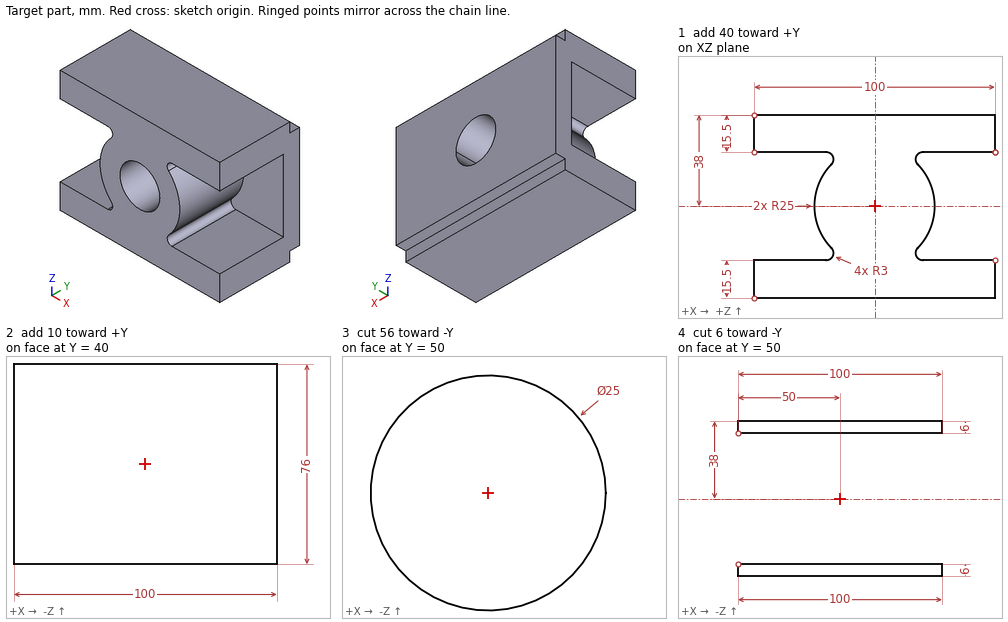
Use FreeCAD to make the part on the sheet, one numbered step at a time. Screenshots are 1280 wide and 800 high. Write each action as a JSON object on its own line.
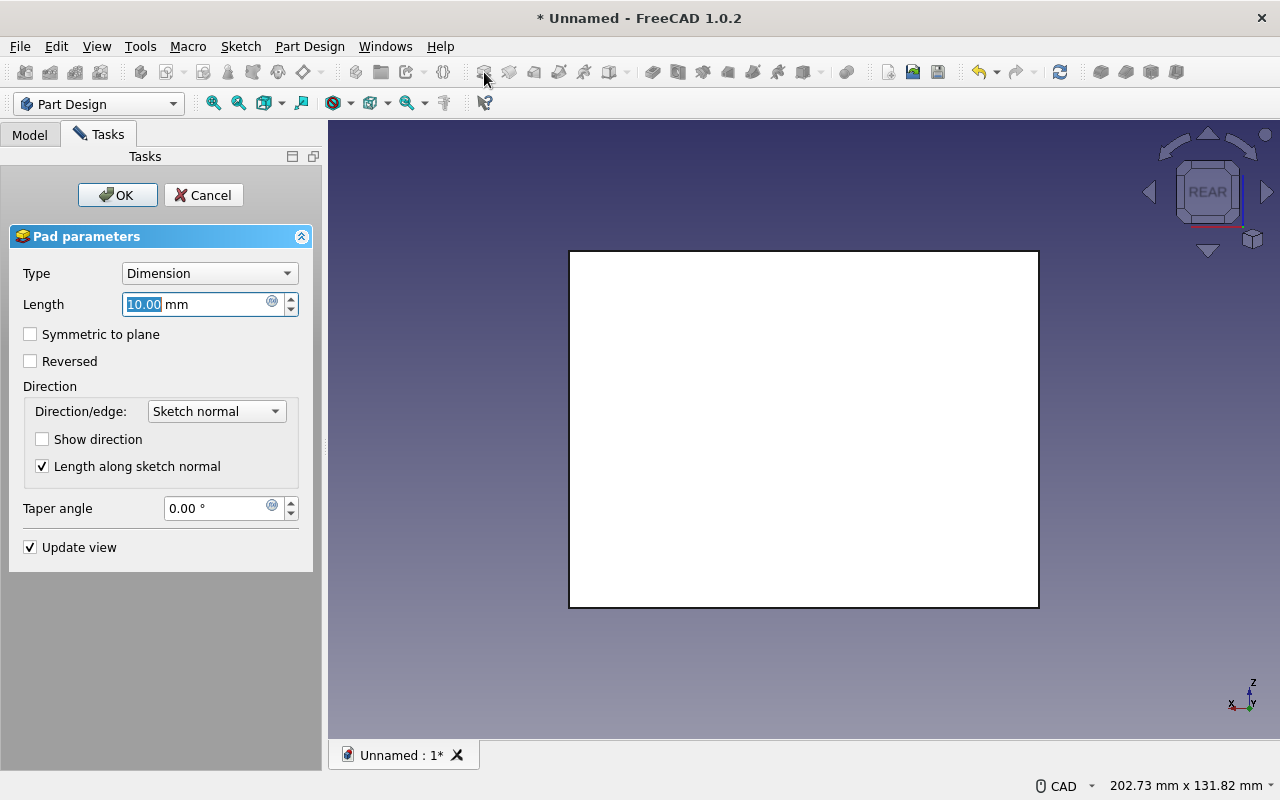
{"action": "type", "text": "10"}
{"action": "key", "text": "Tab"}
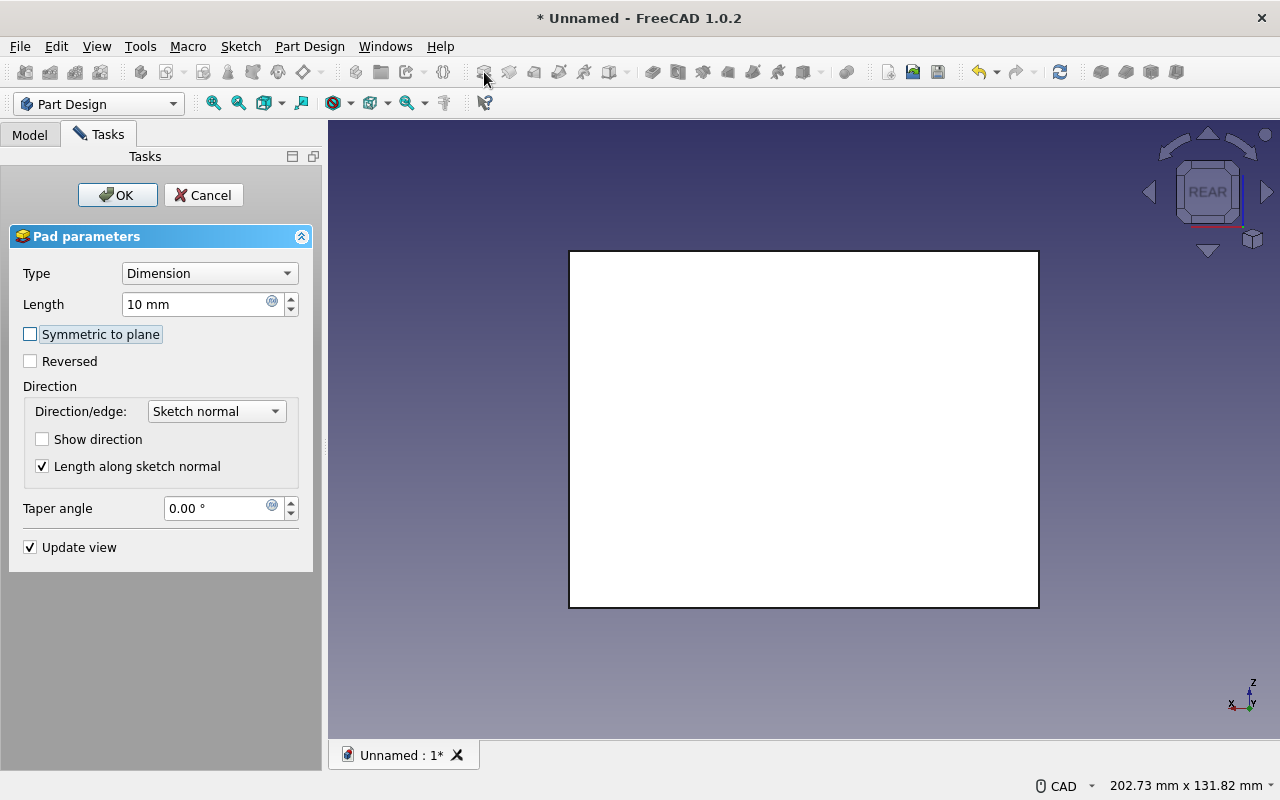
{"action": "left_click", "coordinate": [118, 195]}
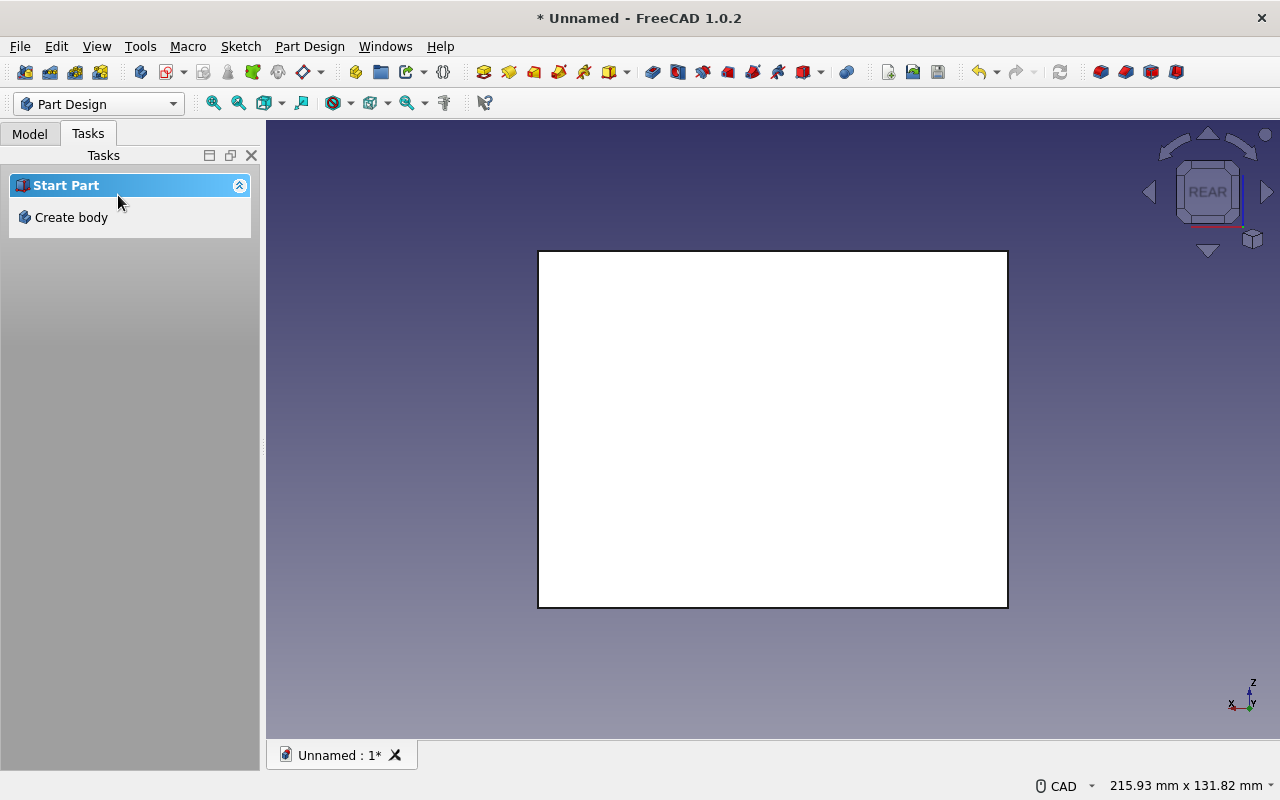
{"action": "left_click", "coordinate": [773, 428]}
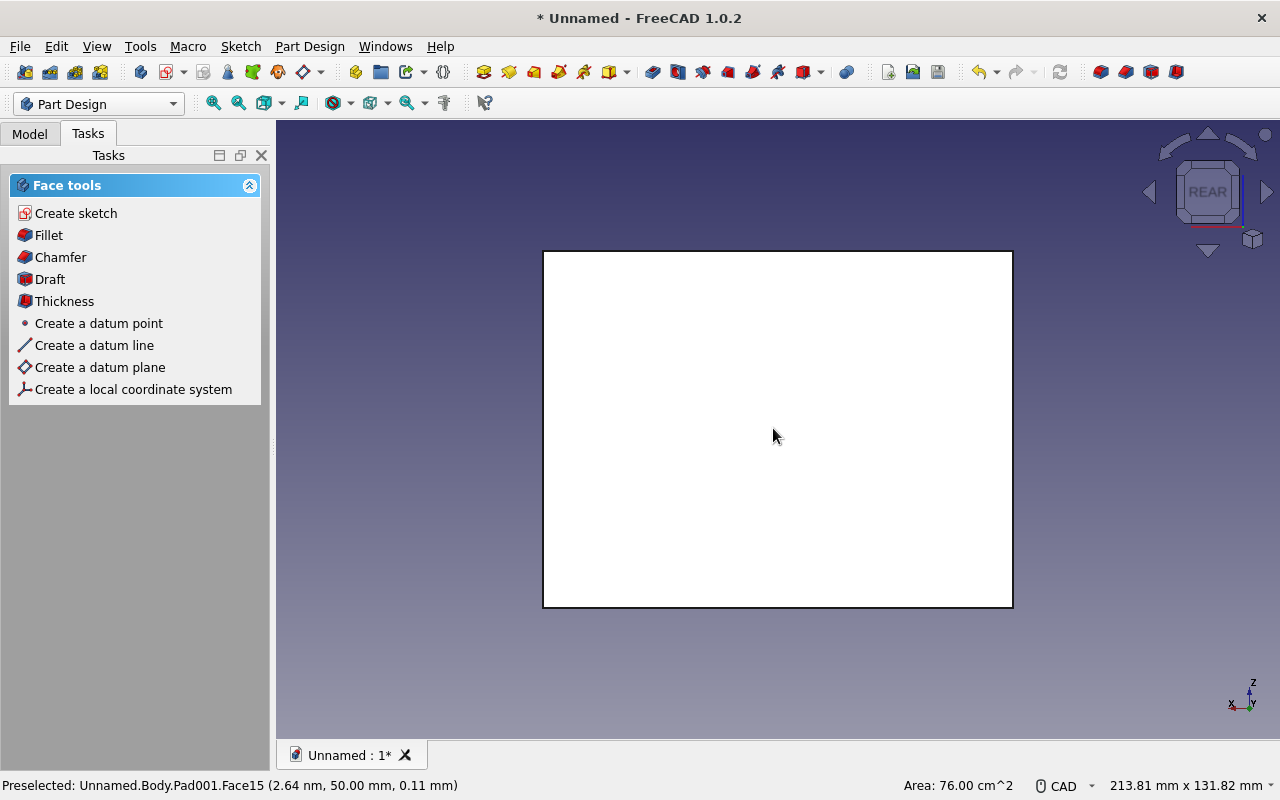
{"action": "left_click", "coordinate": [166, 72]}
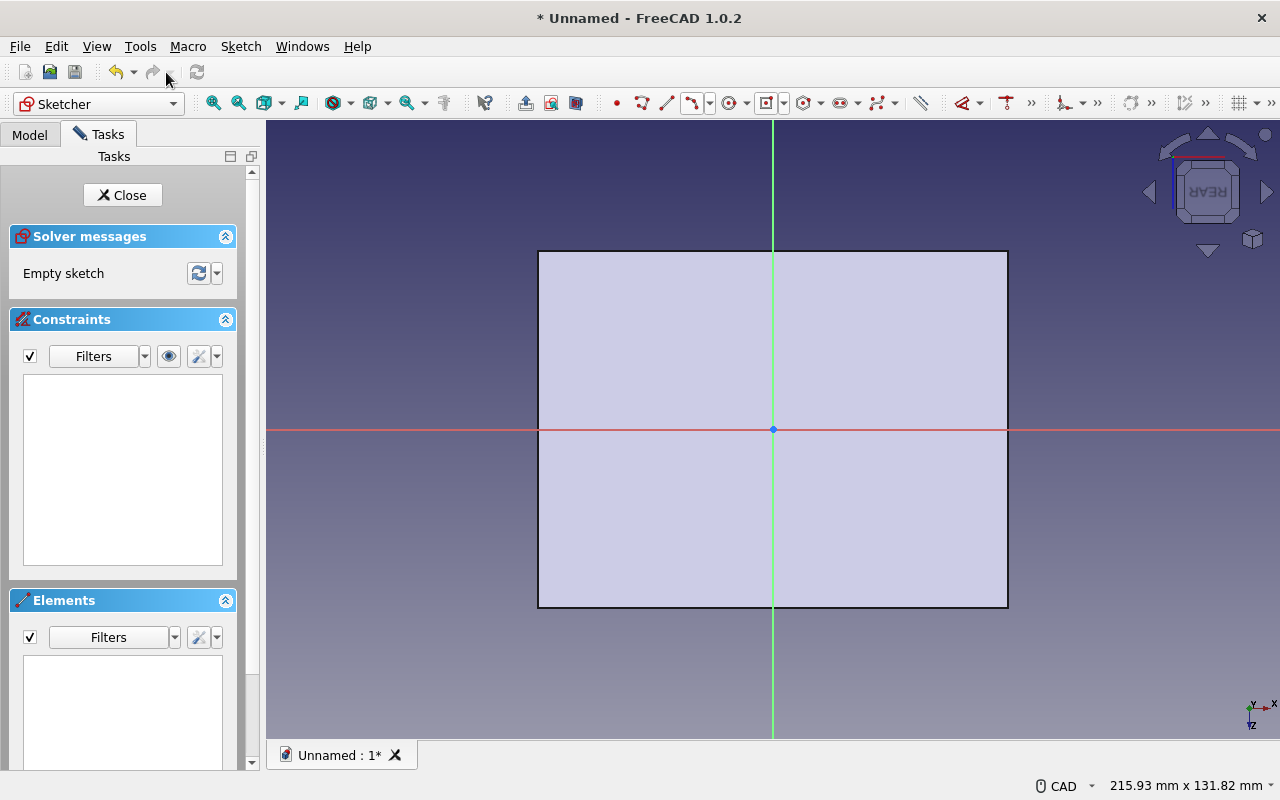
{"action": "scroll", "coordinate": [803, 429], "scroll_direction": "up", "scroll_amount": 6}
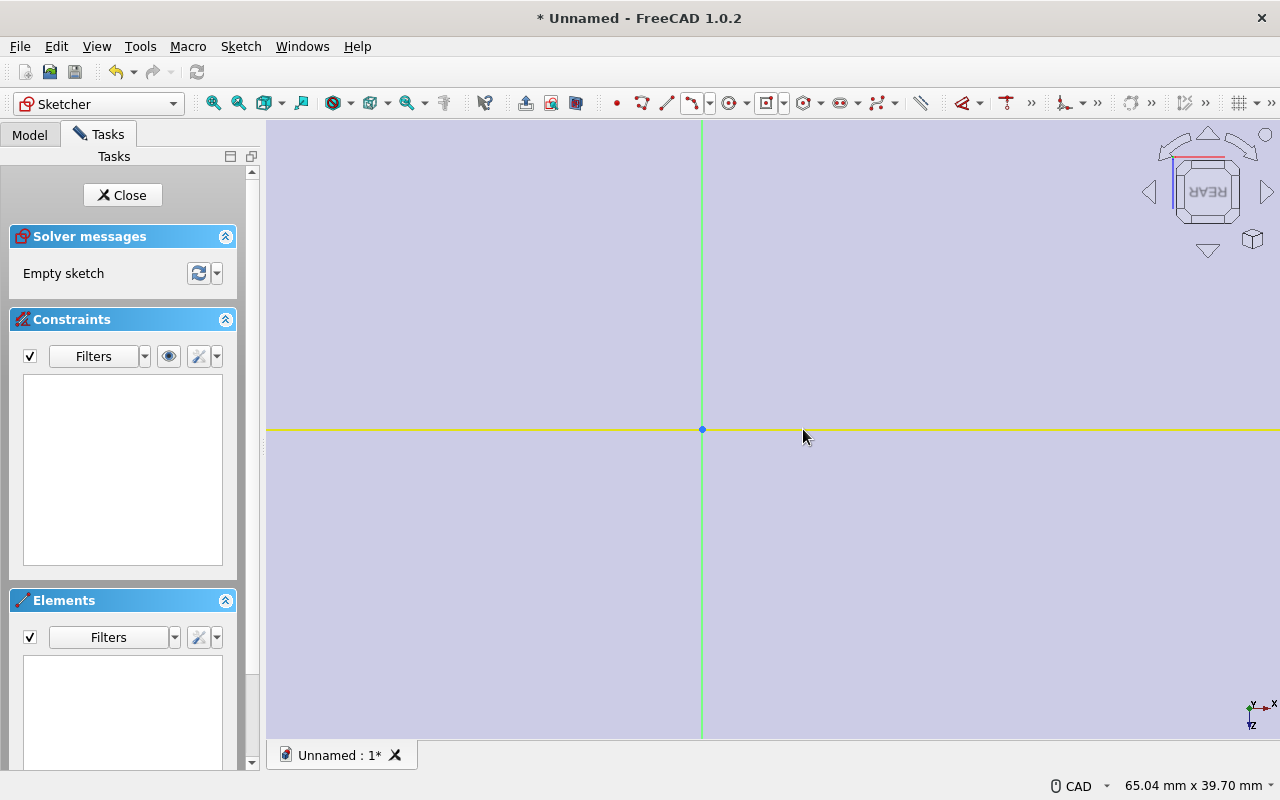
{"action": "left_click", "coordinate": [728, 104]}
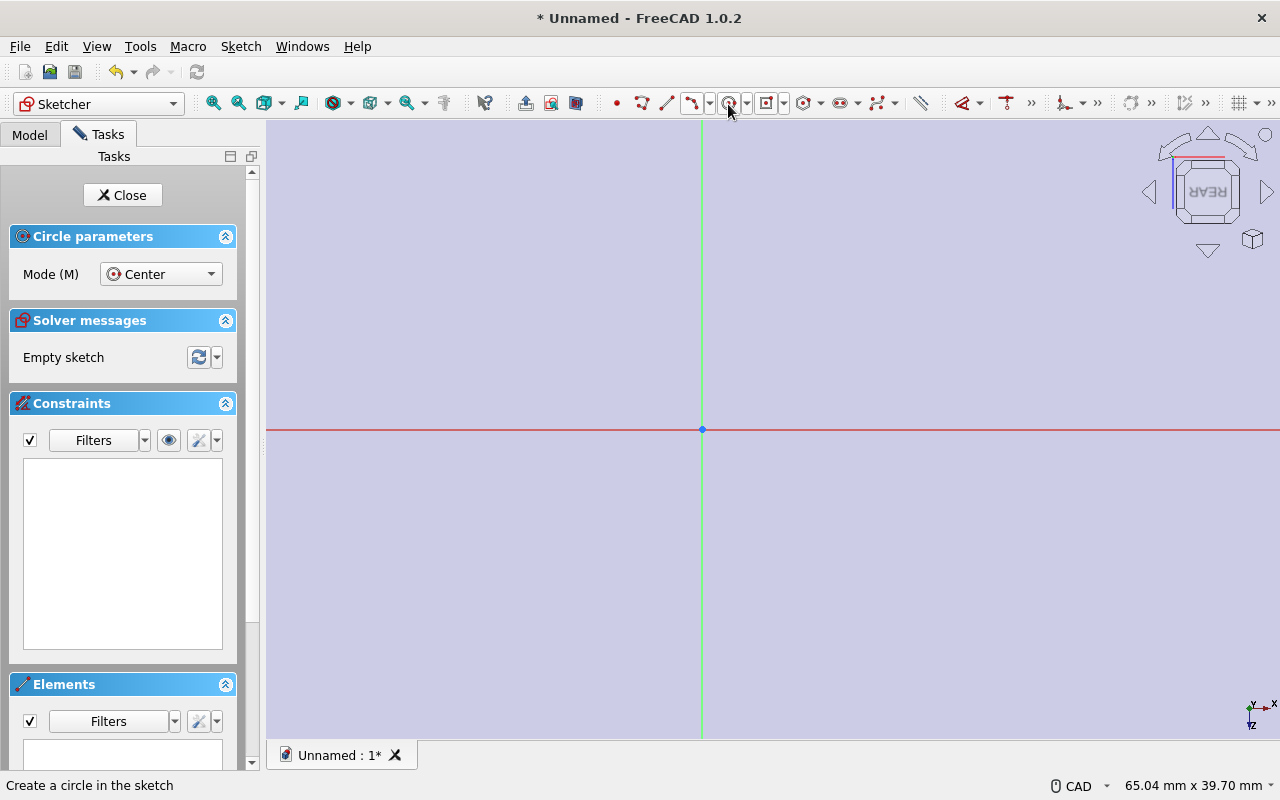
{"action": "left_click", "coordinate": [702, 429]}
{"action": "mouse_move", "coordinate": [840, 292]}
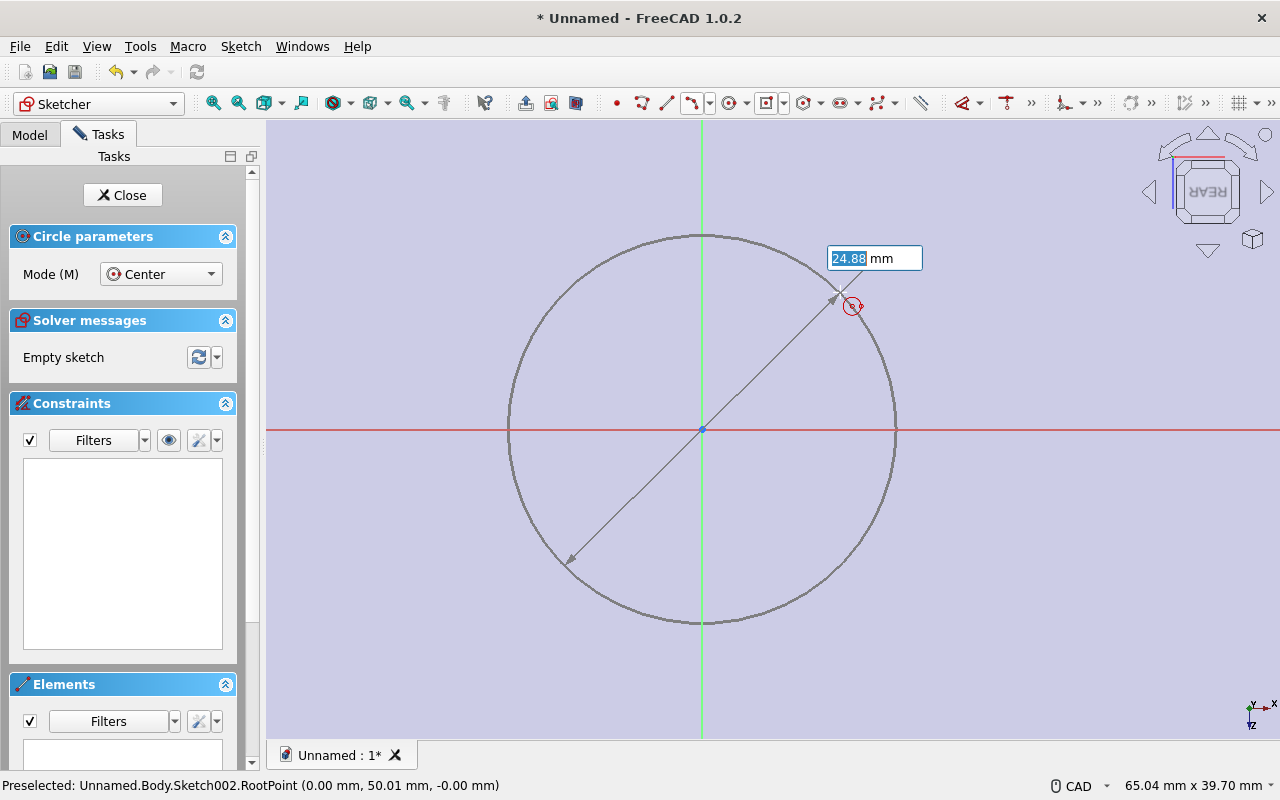
{"action": "type", "text": "25"}
{"action": "key", "text": "Return"}
{"action": "key", "text": "Escape"}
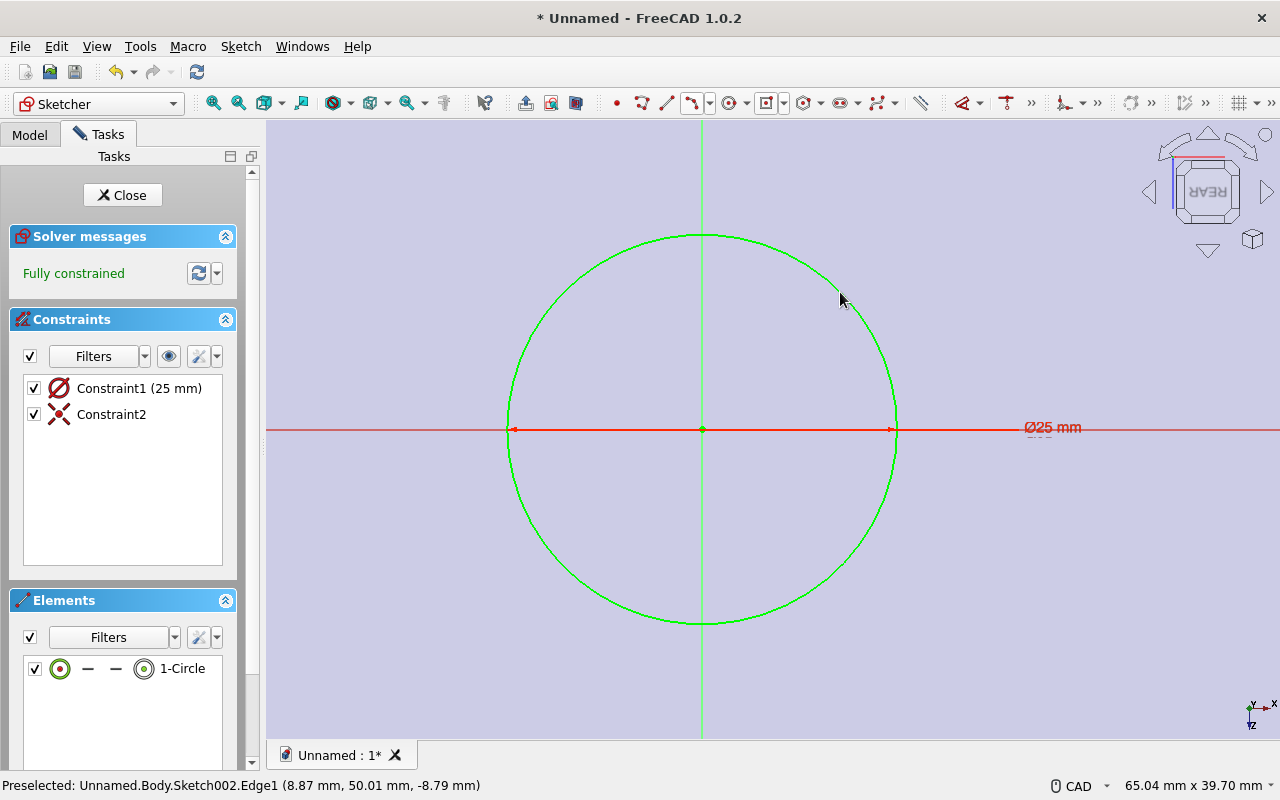
{"action": "left_click", "coordinate": [123, 195]}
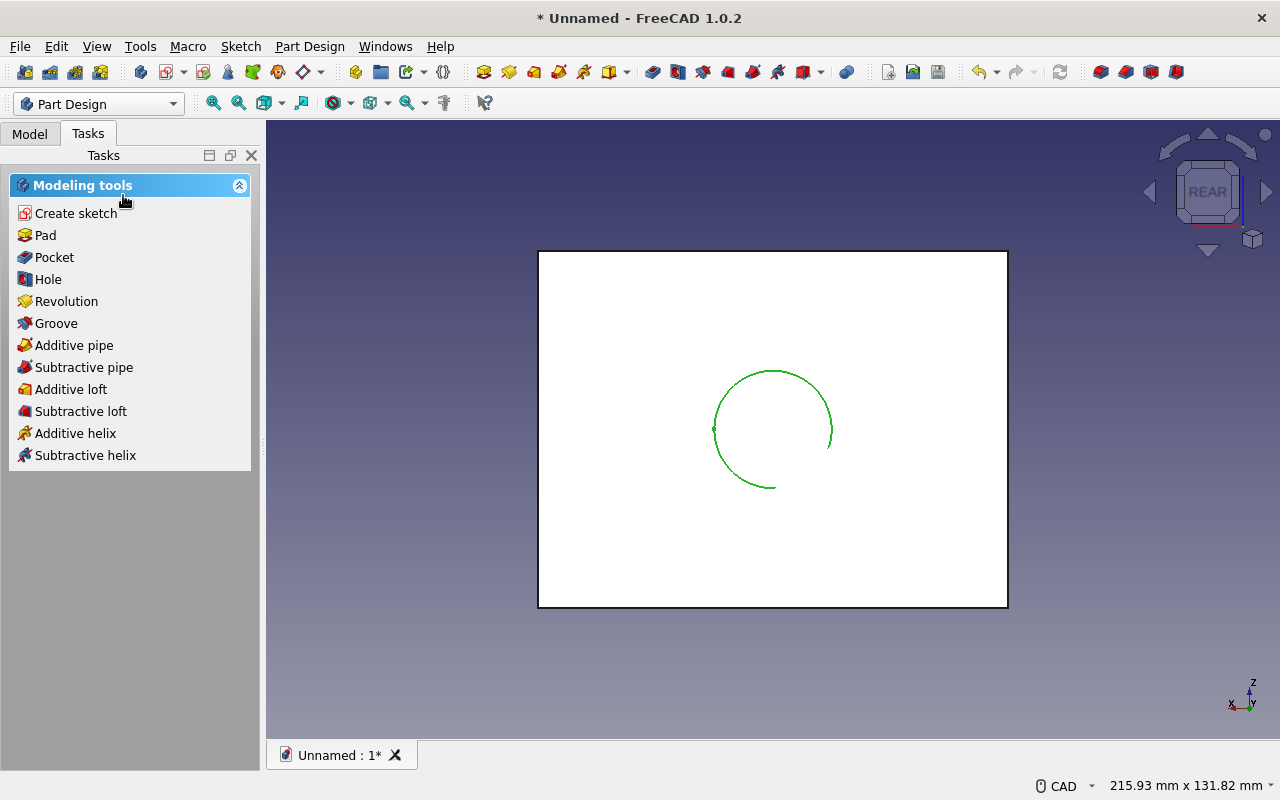
{"action": "left_click", "coordinate": [653, 72]}